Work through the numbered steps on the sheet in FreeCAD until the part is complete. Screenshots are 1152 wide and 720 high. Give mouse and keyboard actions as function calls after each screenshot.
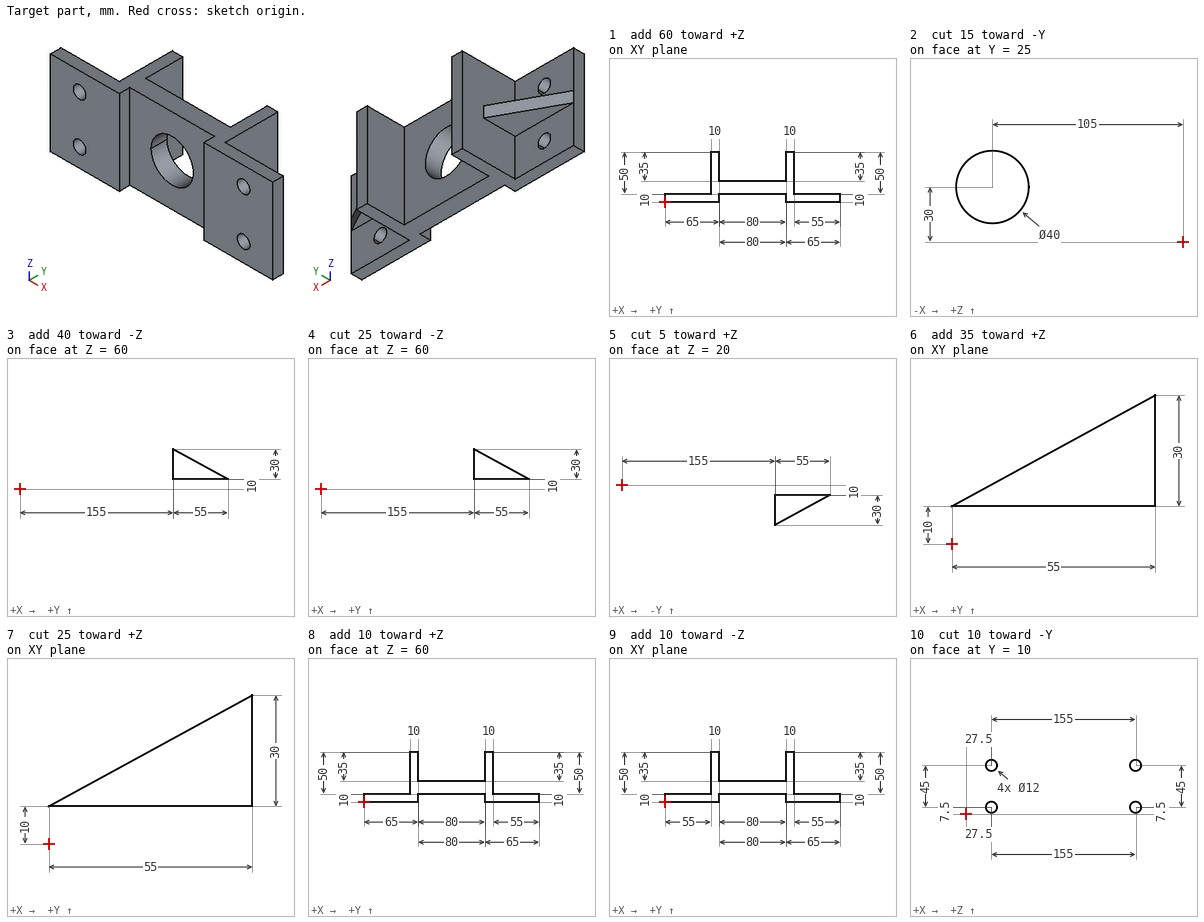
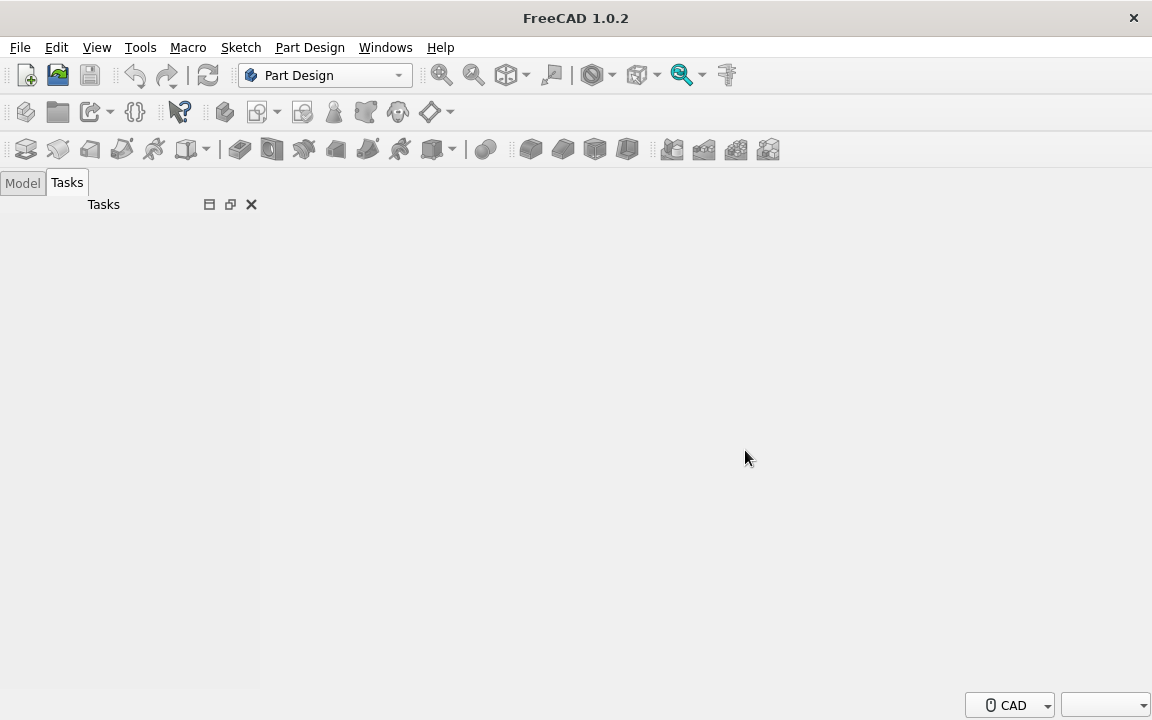
key(ctrl+n)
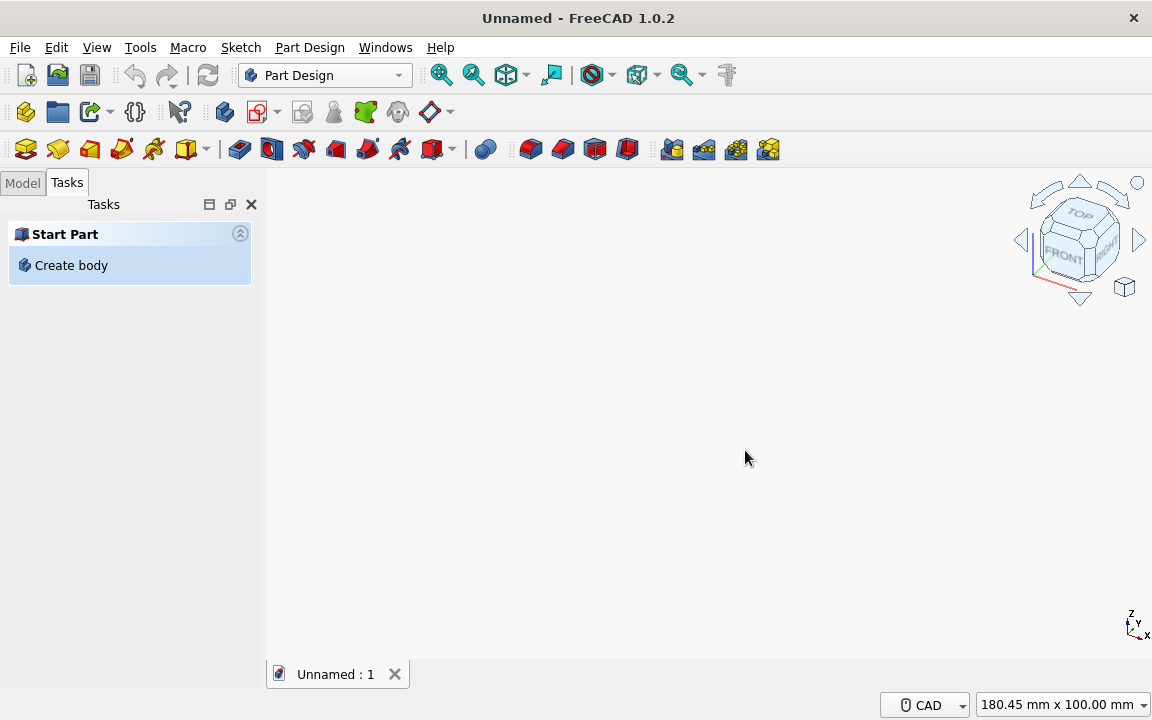
click(258, 112)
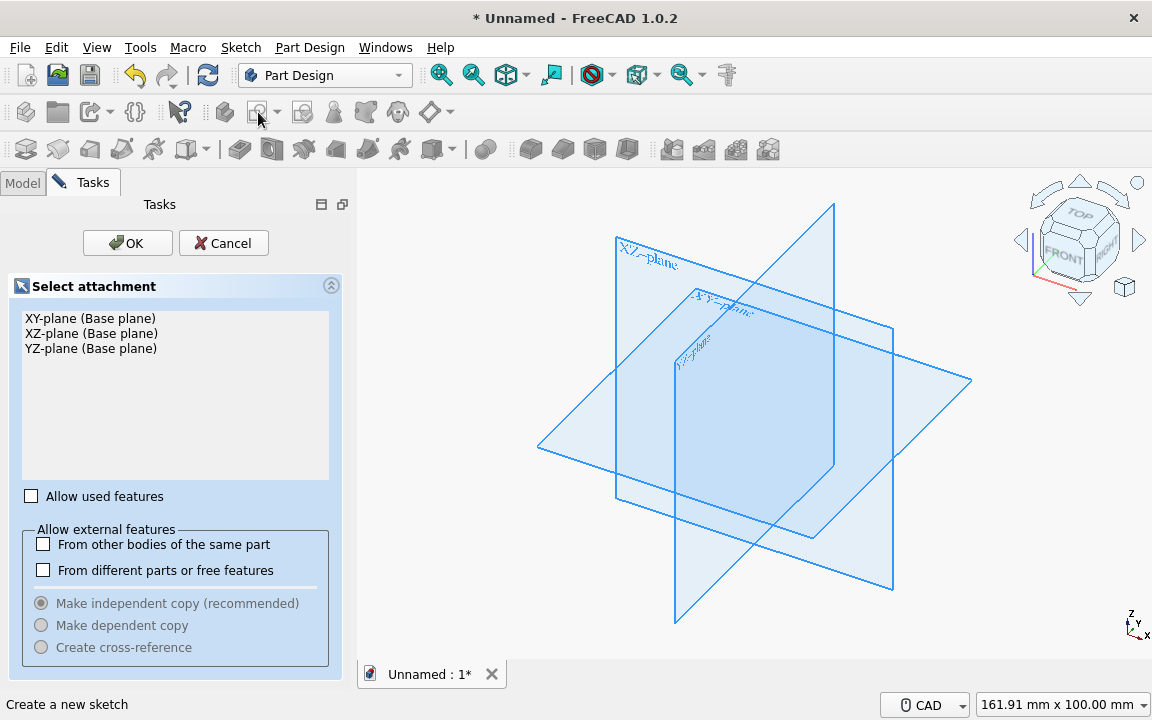
click(82, 318)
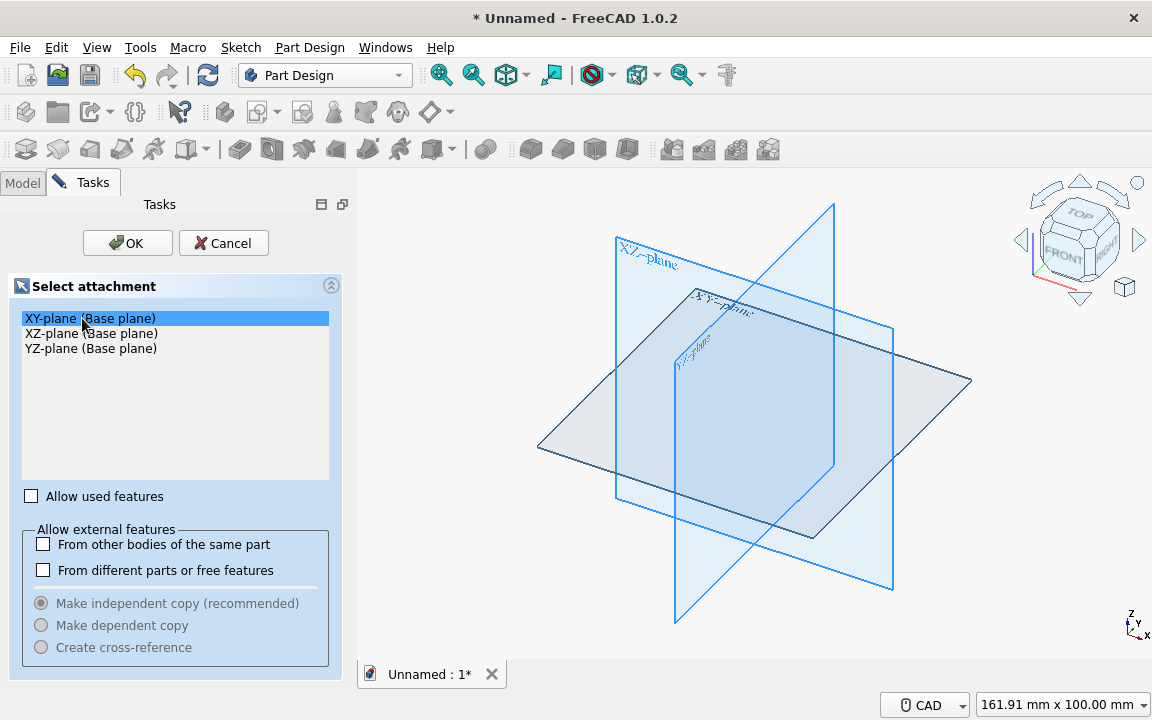
click(128, 243)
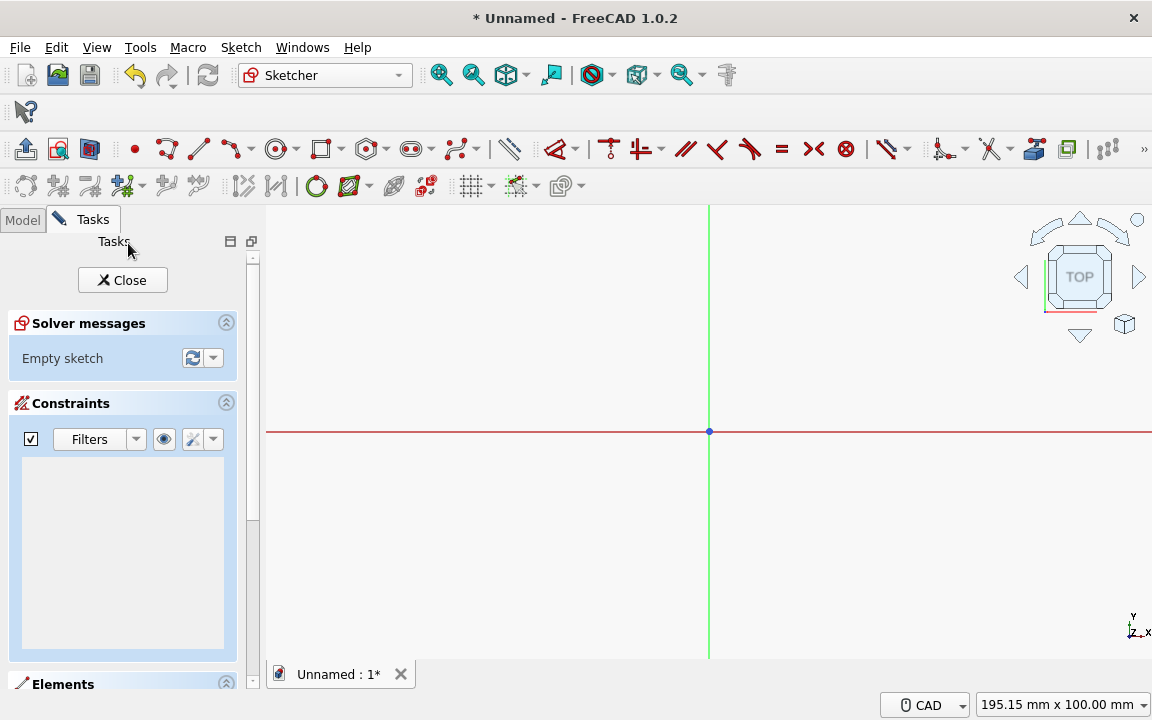
scroll(294, 543, down, 4)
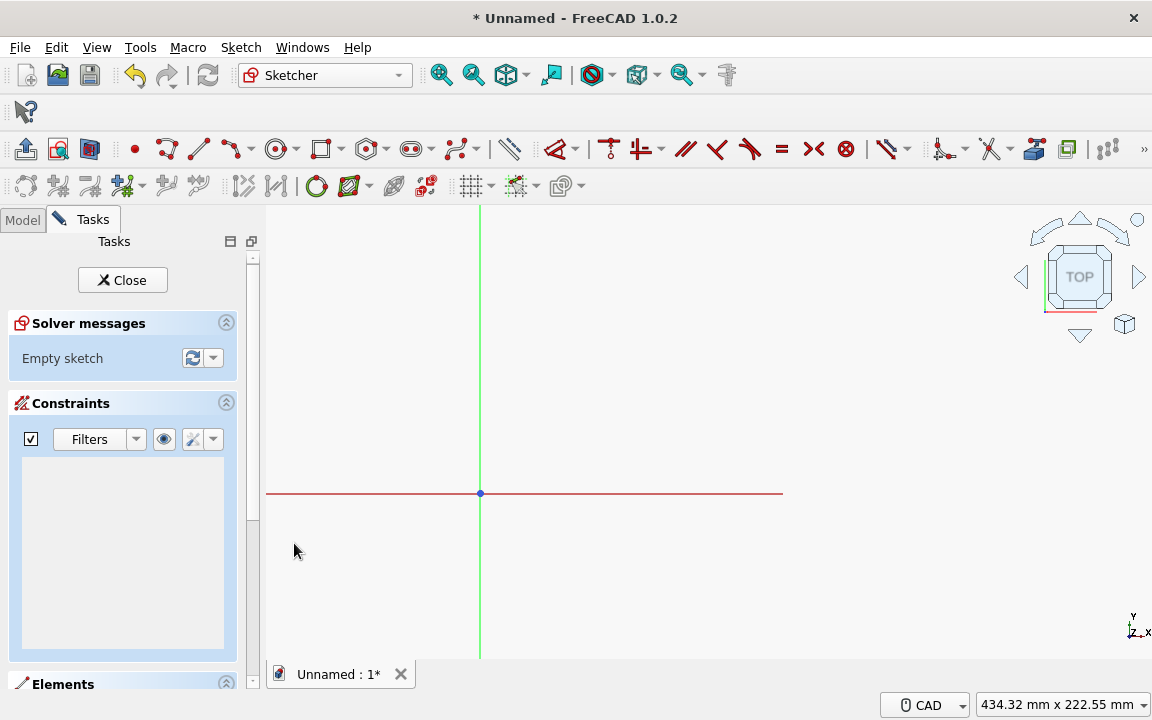
key(g)
key(m)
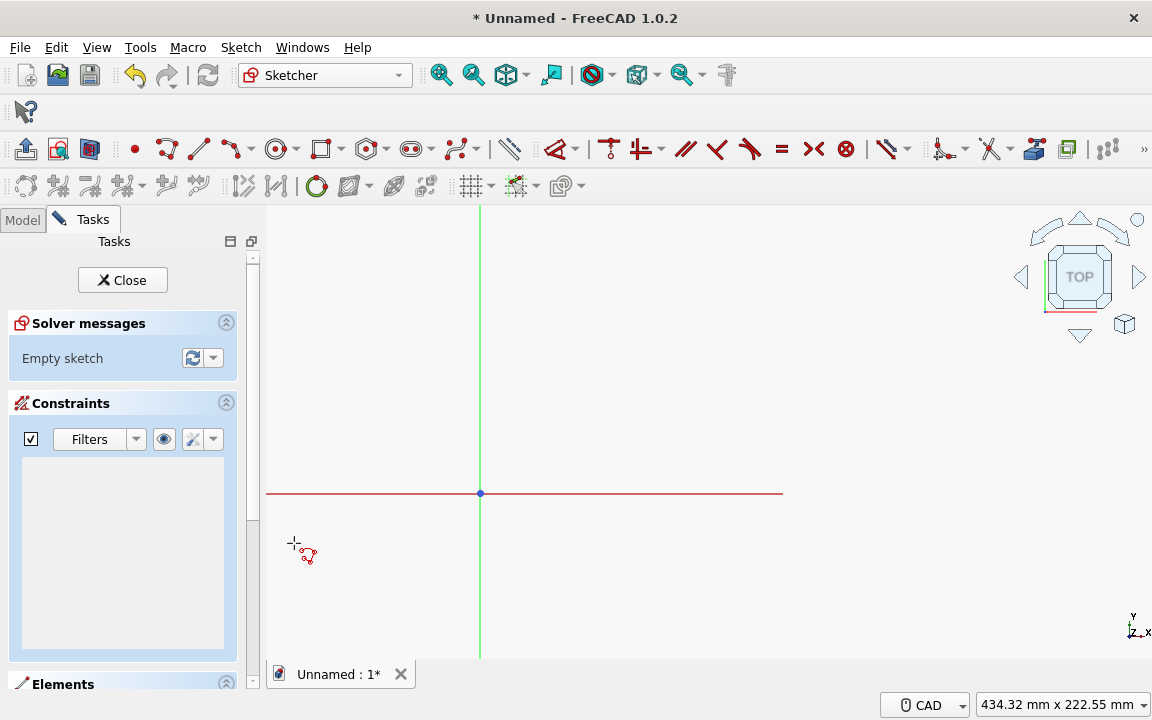
click(480, 494)
click(613, 485)
click(613, 473)
click(776, 473)
click(776, 494)
click(909, 485)
click(909, 473)
click(797, 473)
click(797, 371)
click(776, 371)
click(776, 443)
click(613, 443)
click(613, 371)
click(593, 371)
click(593, 473)
click(489, 473)
click(480, 494)
key(Escape)
key(Escape)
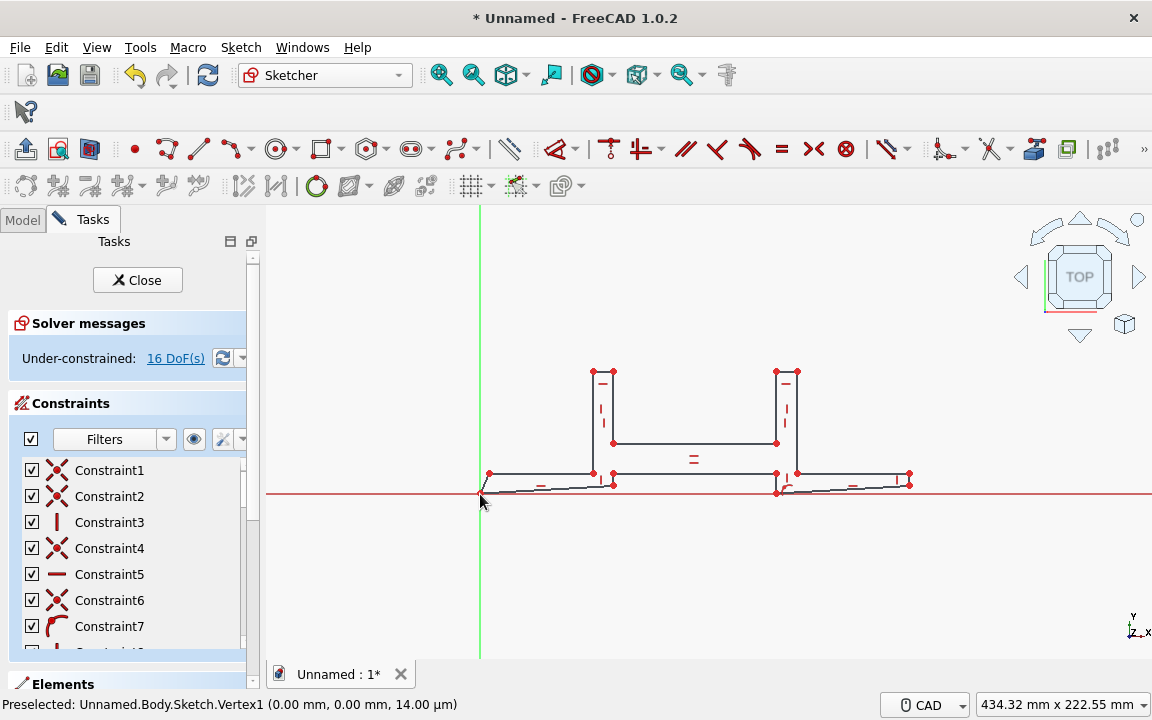
click(520, 491)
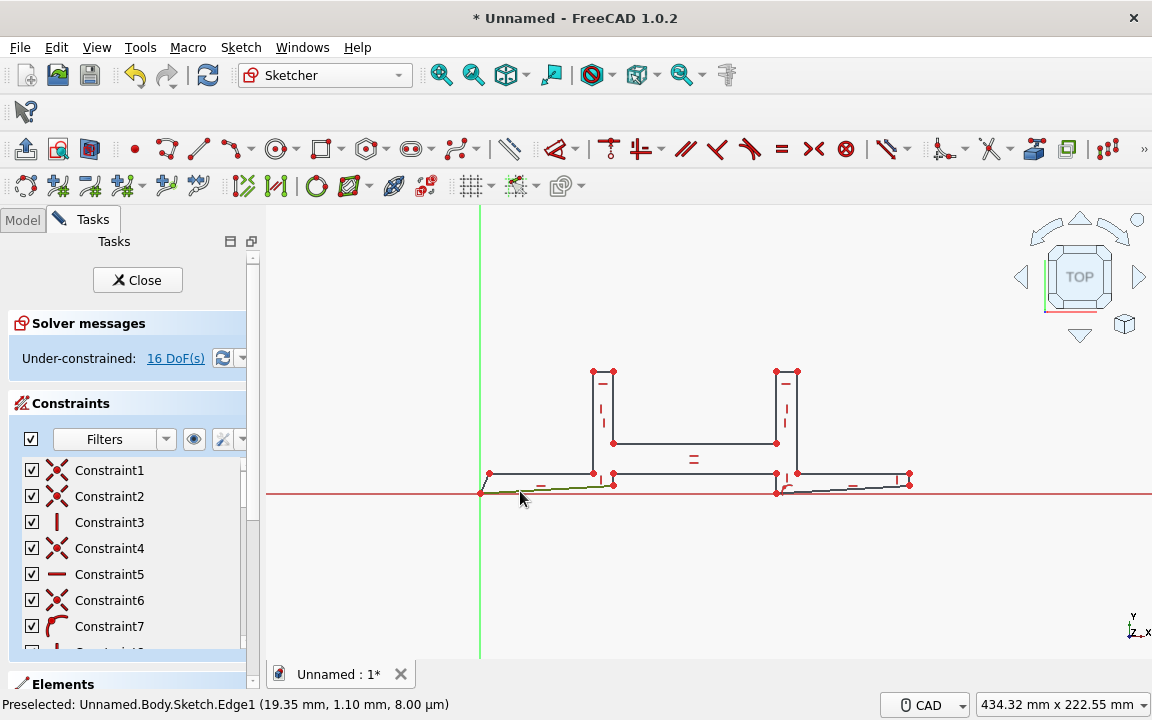
key(h)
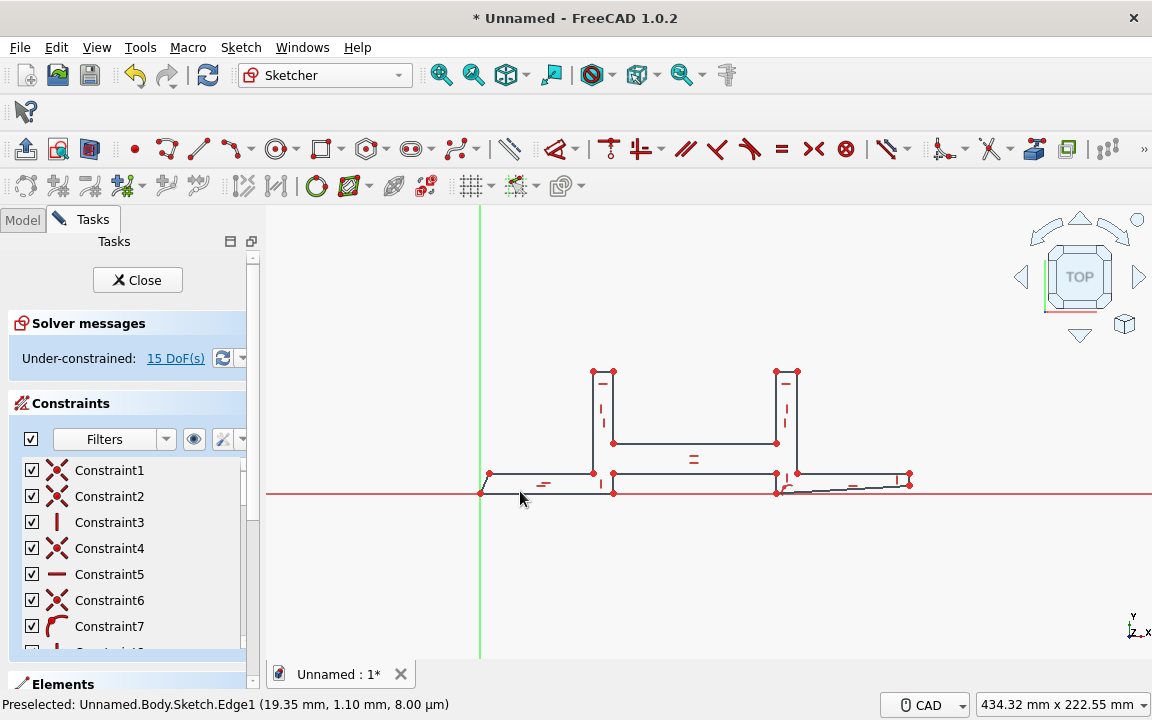
click(816, 491)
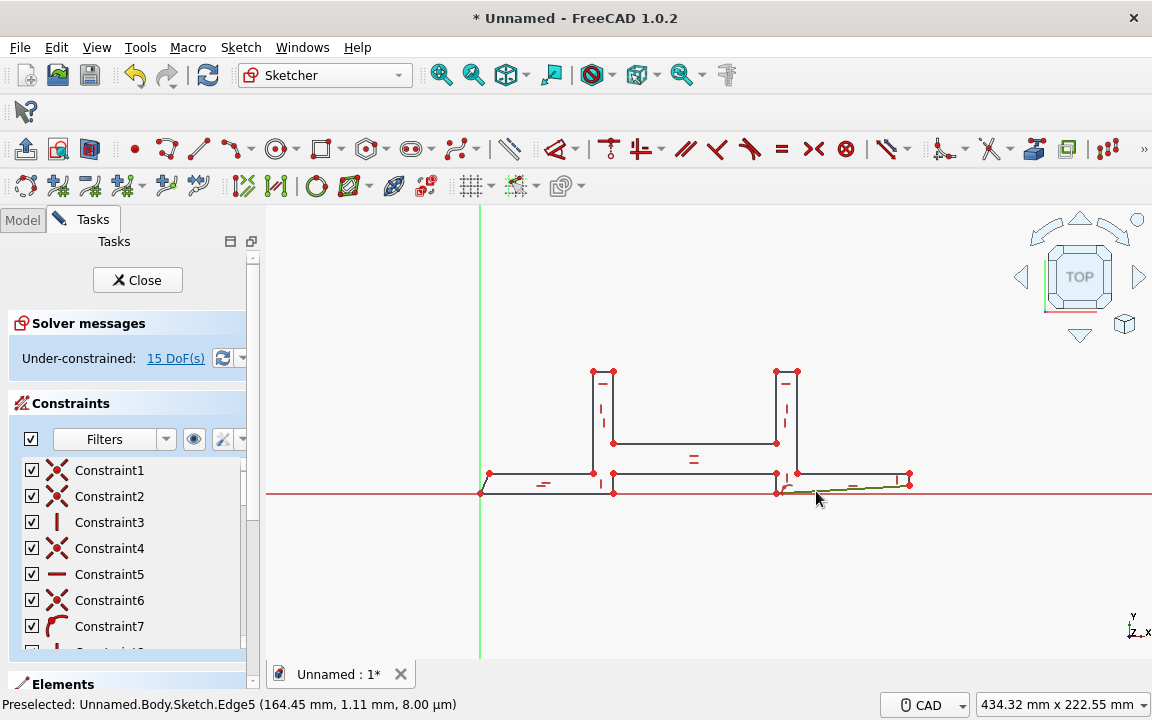
key(h)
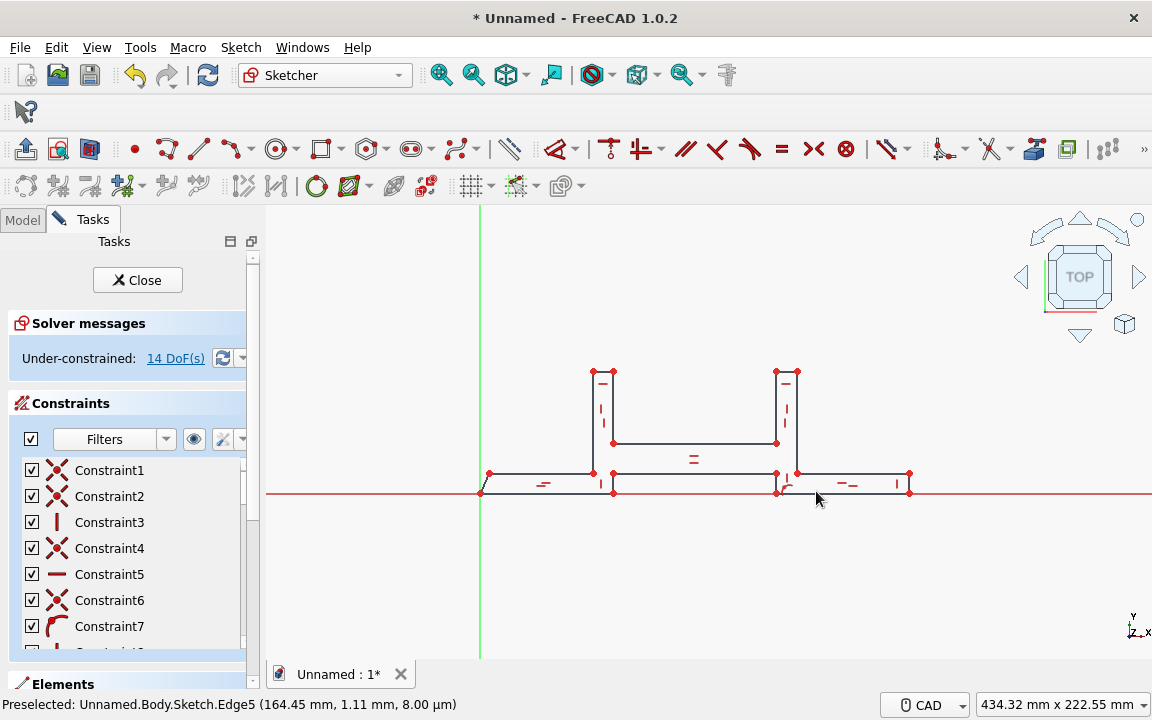
scroll(484, 486, up, 3)